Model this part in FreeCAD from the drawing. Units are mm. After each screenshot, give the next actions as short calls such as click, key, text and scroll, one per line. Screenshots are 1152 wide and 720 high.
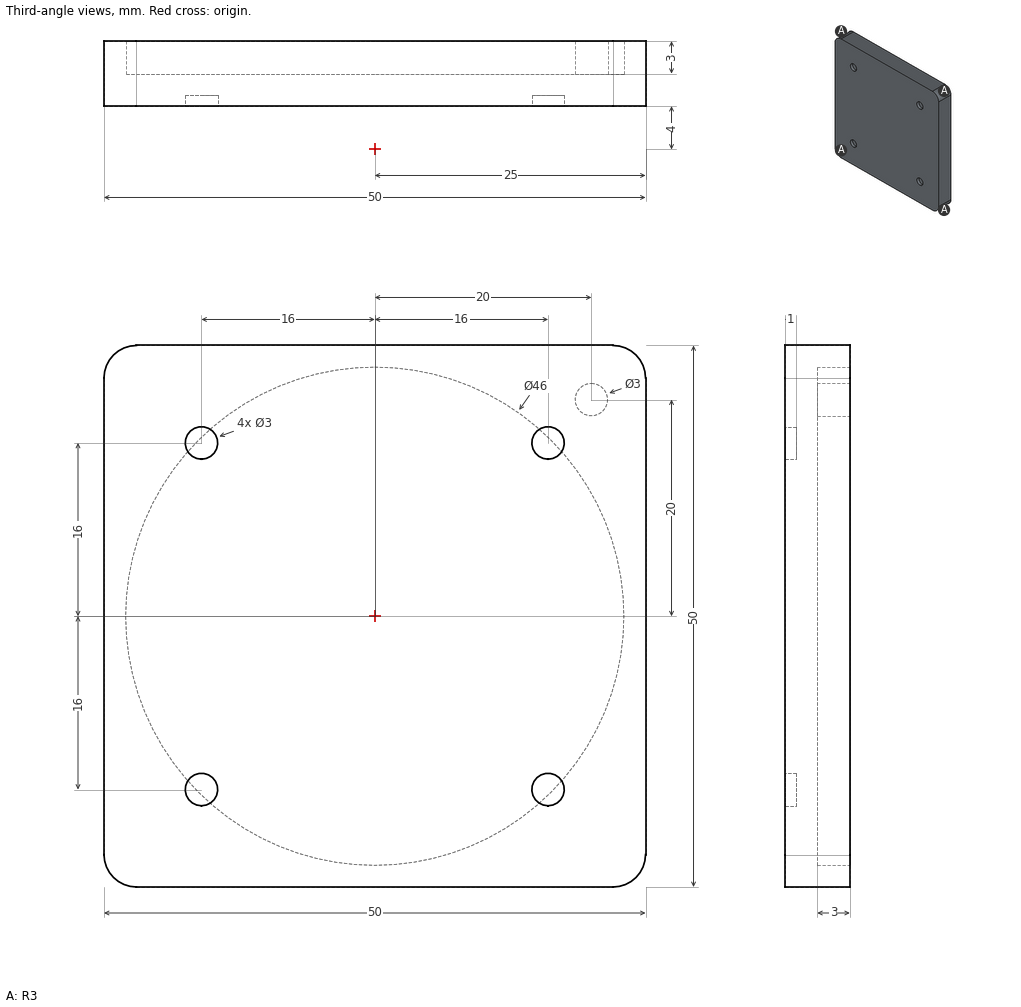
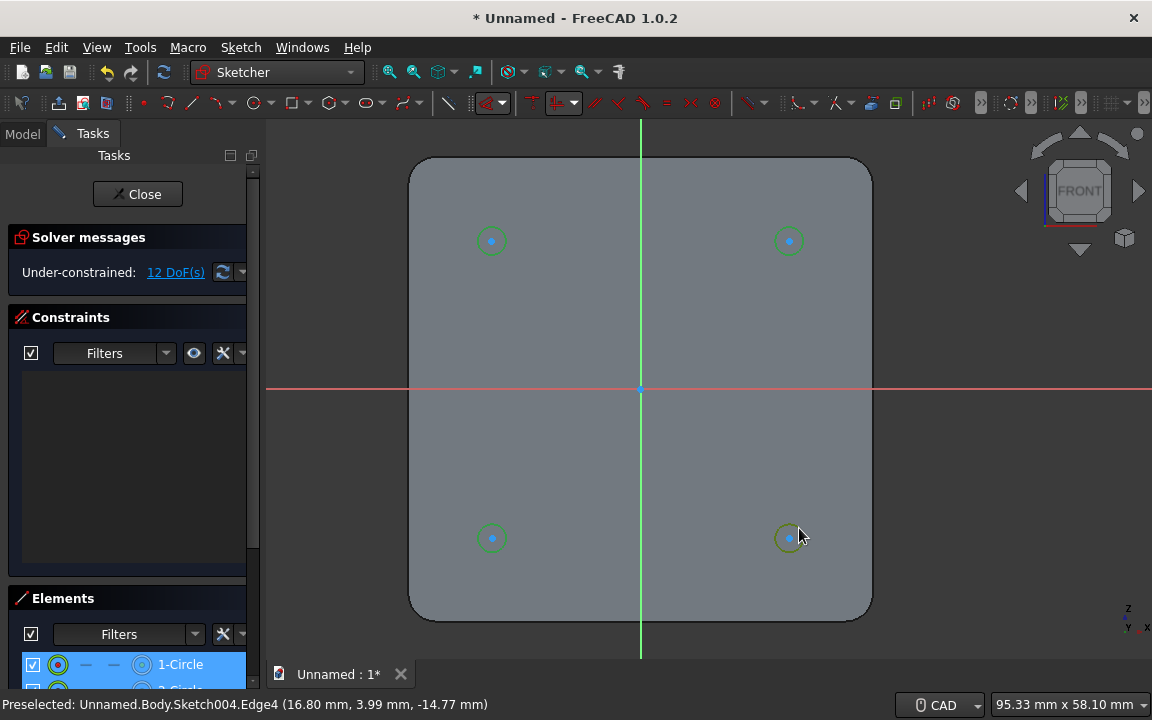
click(668, 104)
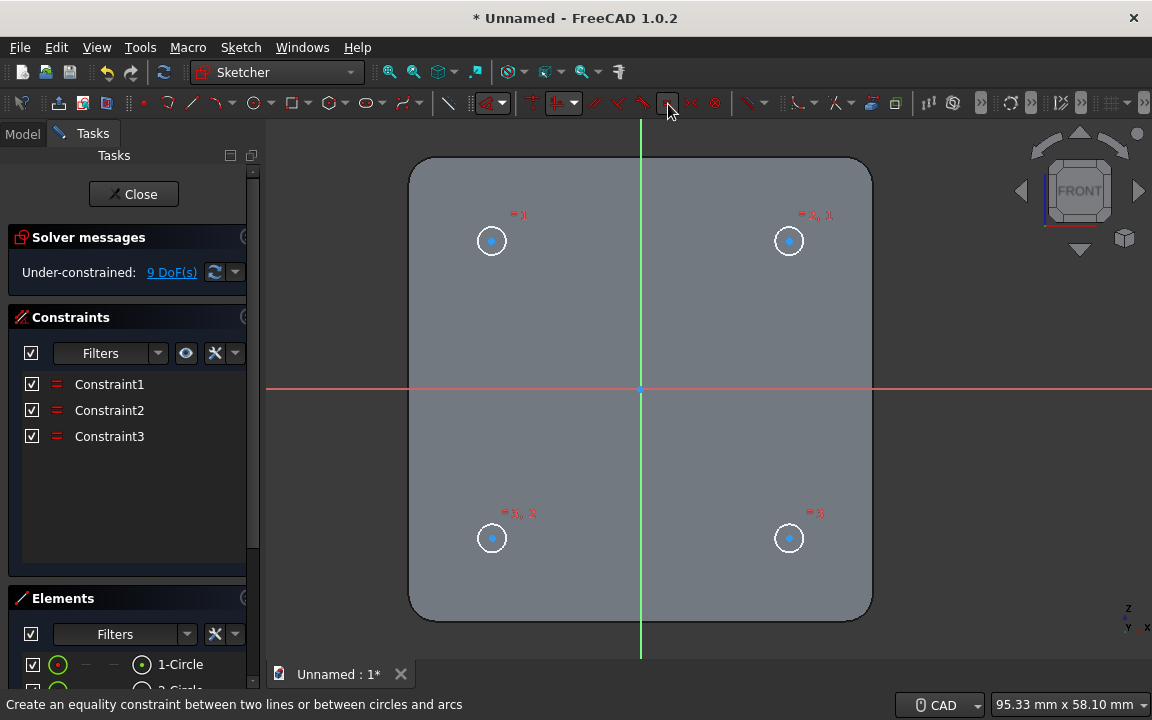
click(492, 241)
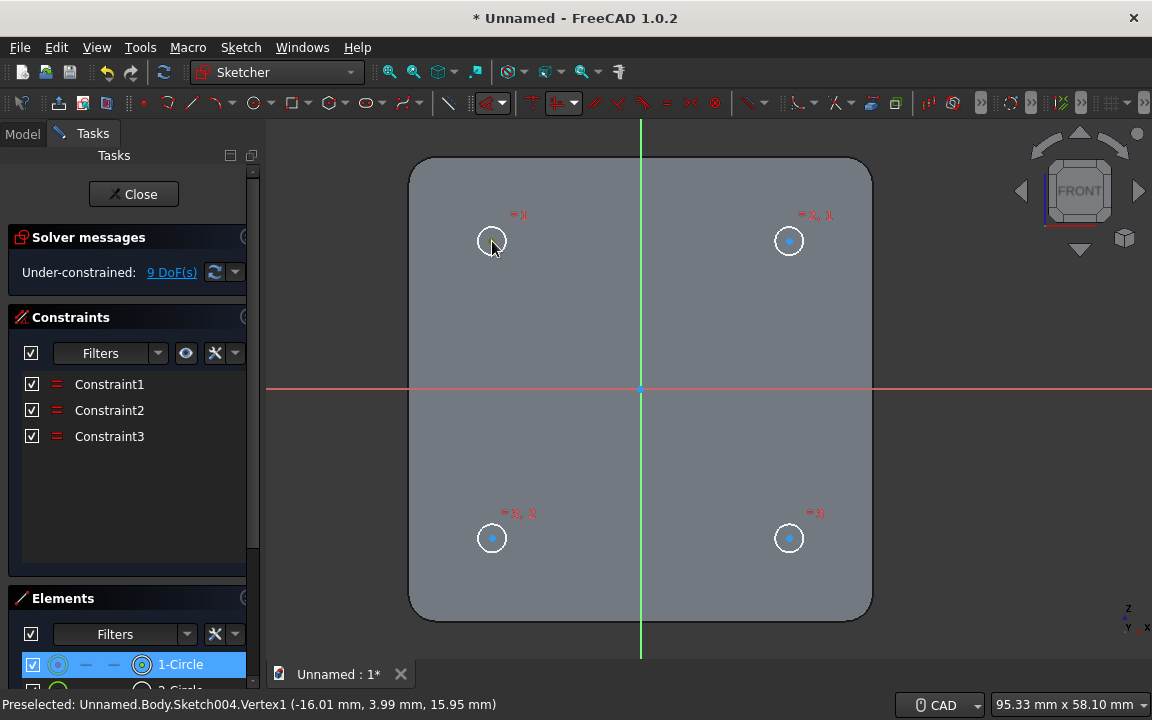
click(789, 241)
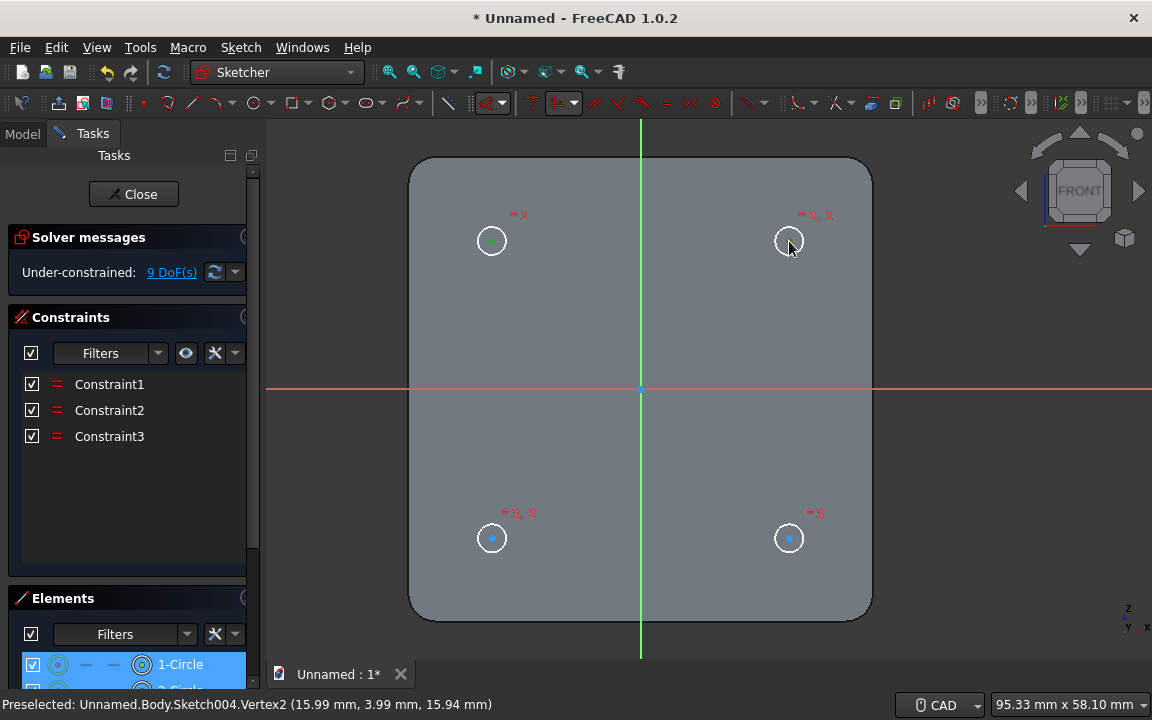
key(h)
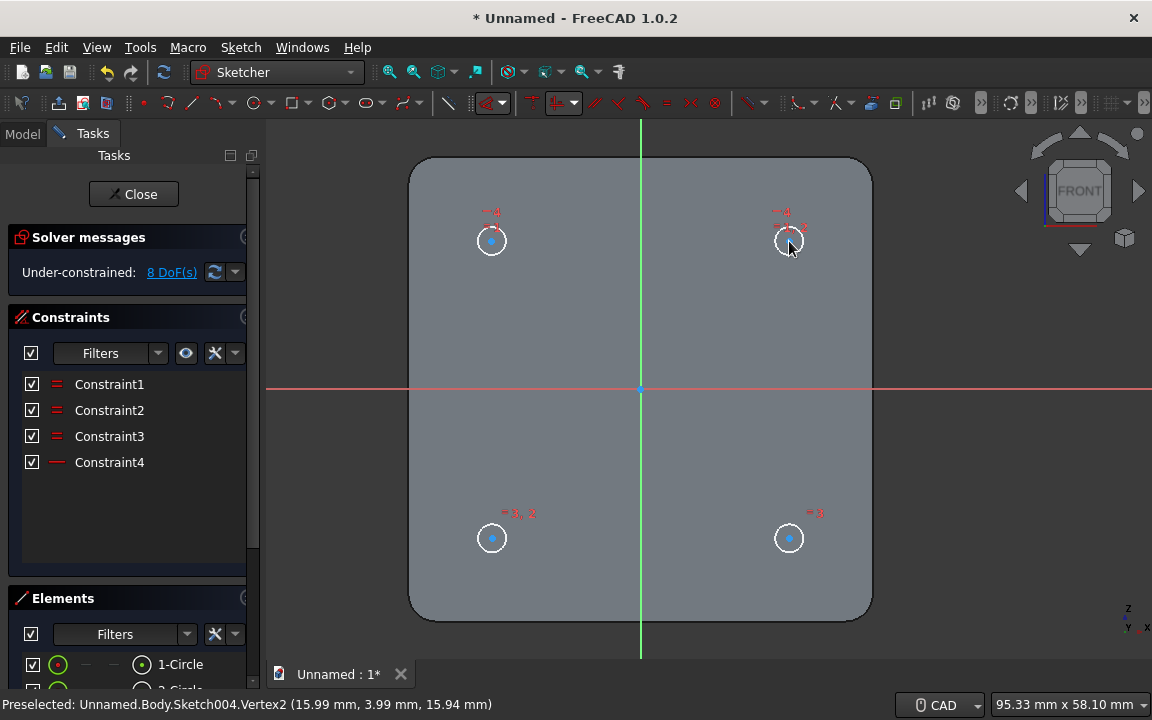
click(492, 241)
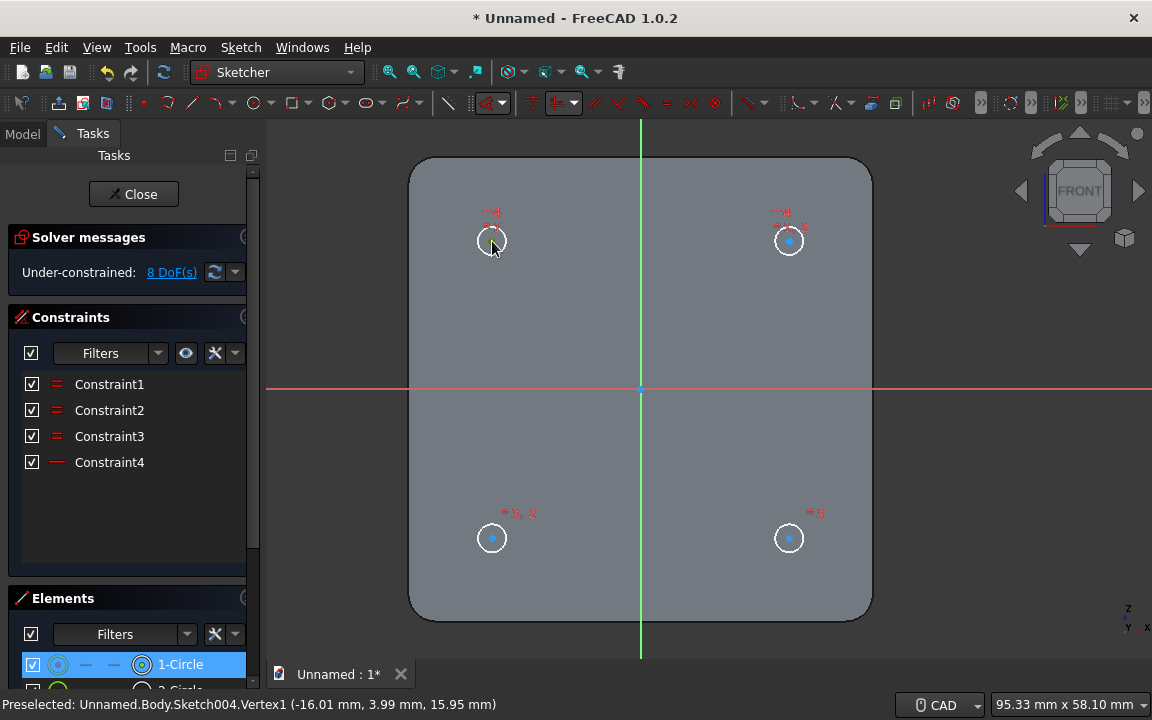
click(492, 538)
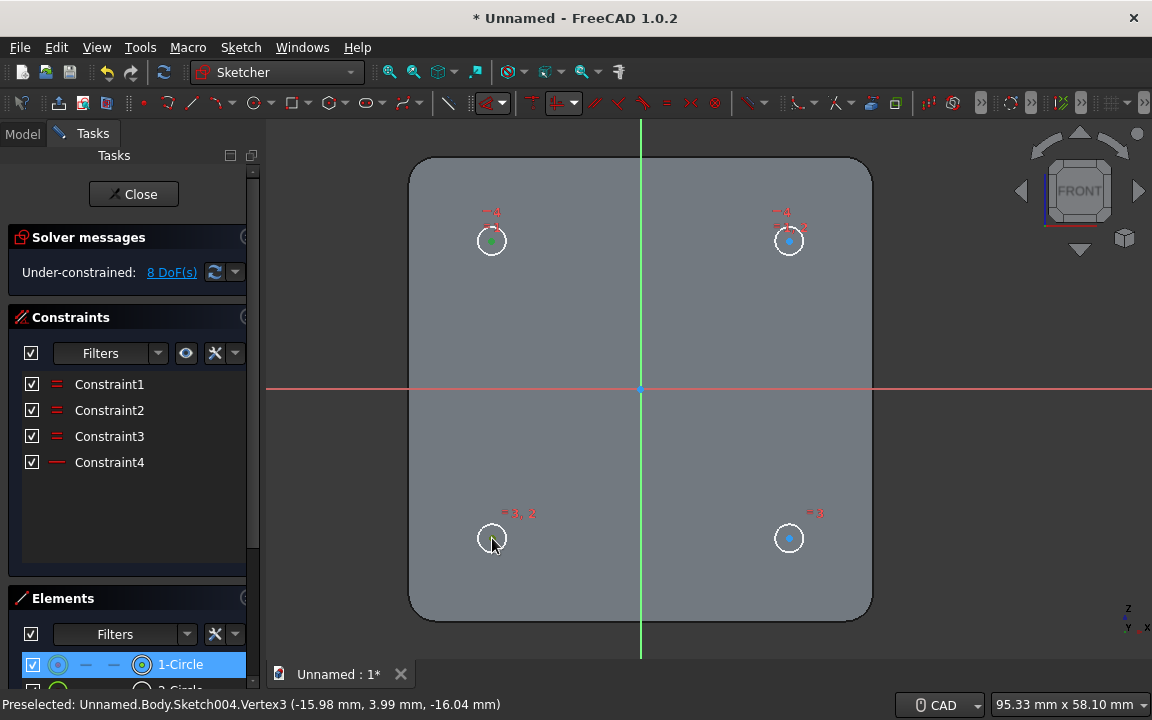
key(v)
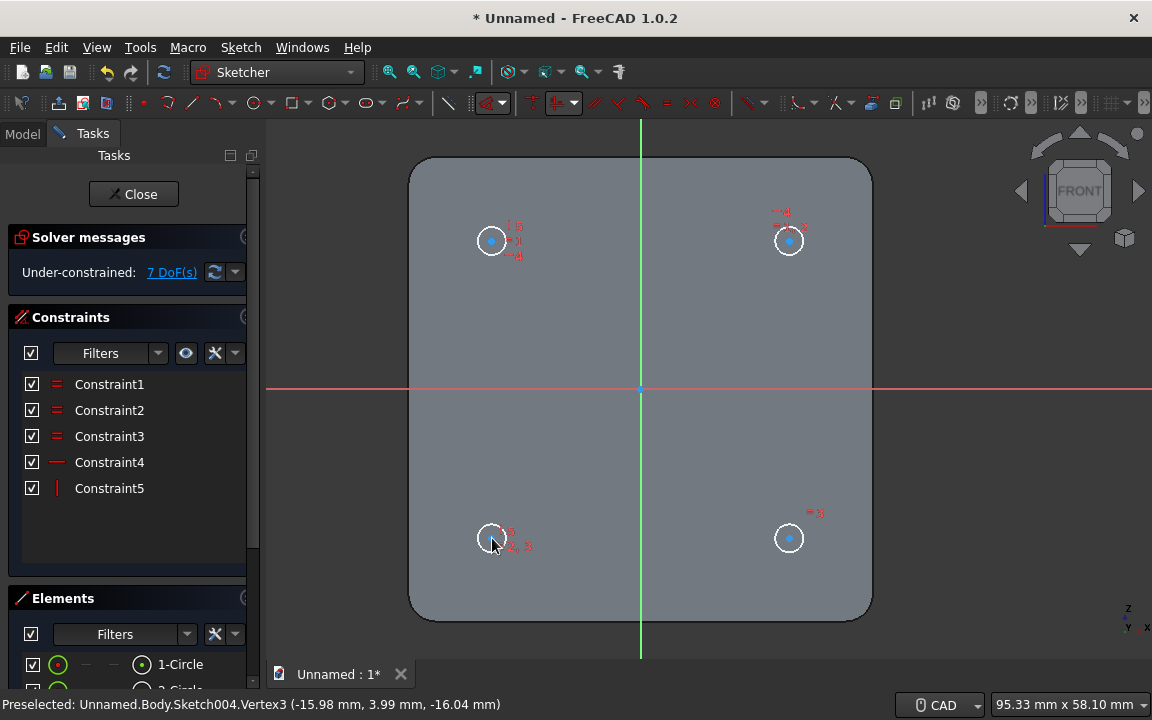
click(789, 241)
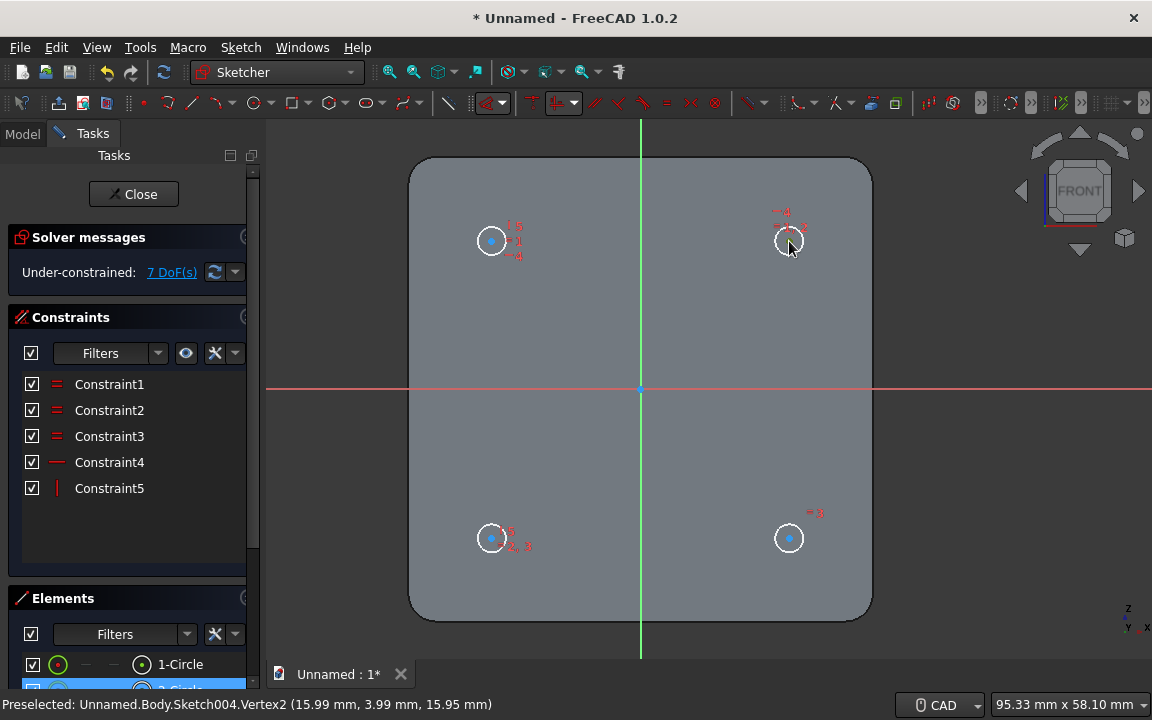
click(789, 538)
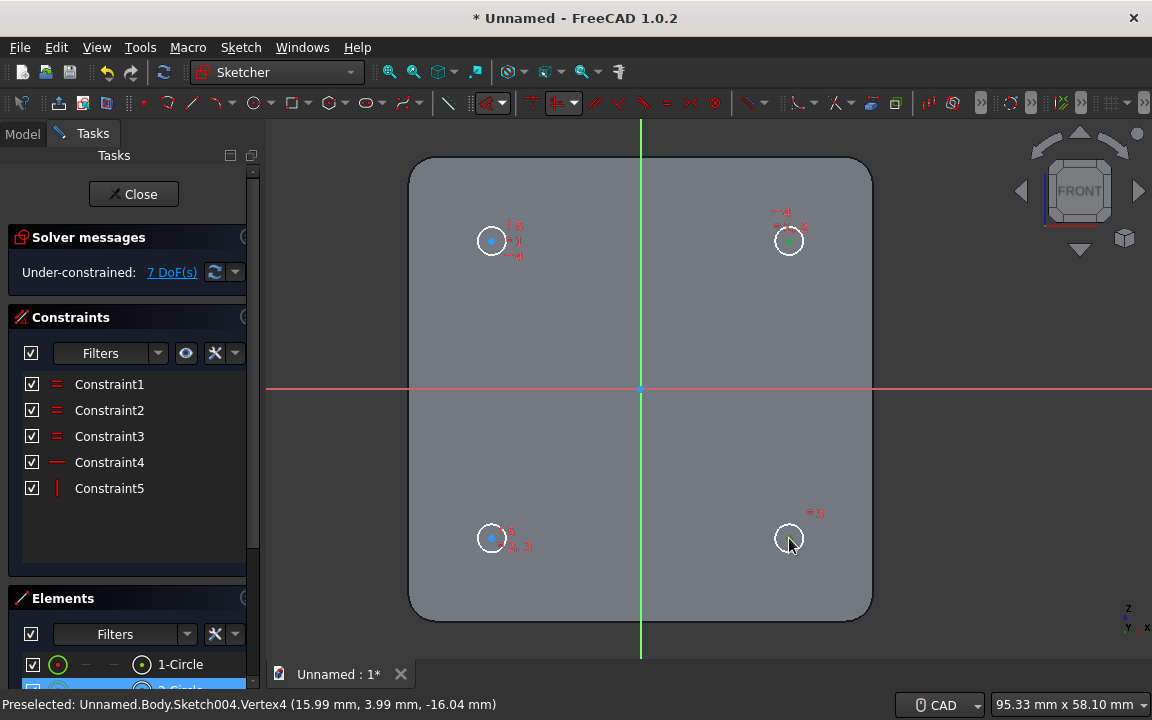
key(v)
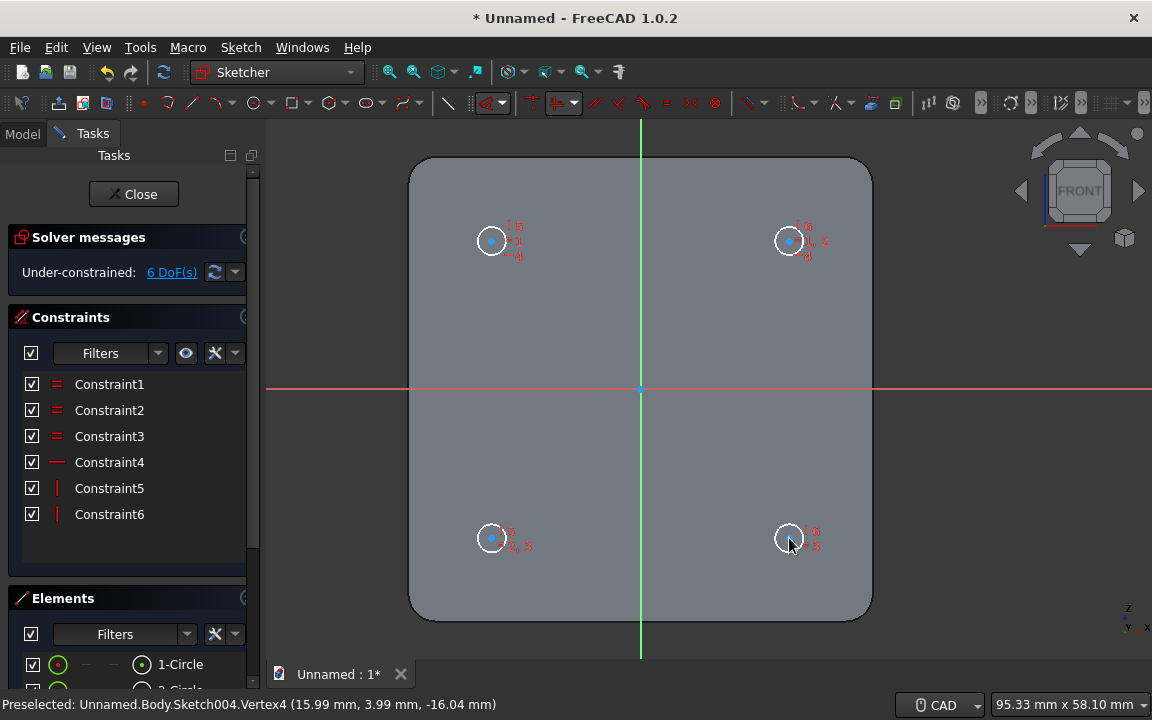
click(492, 538)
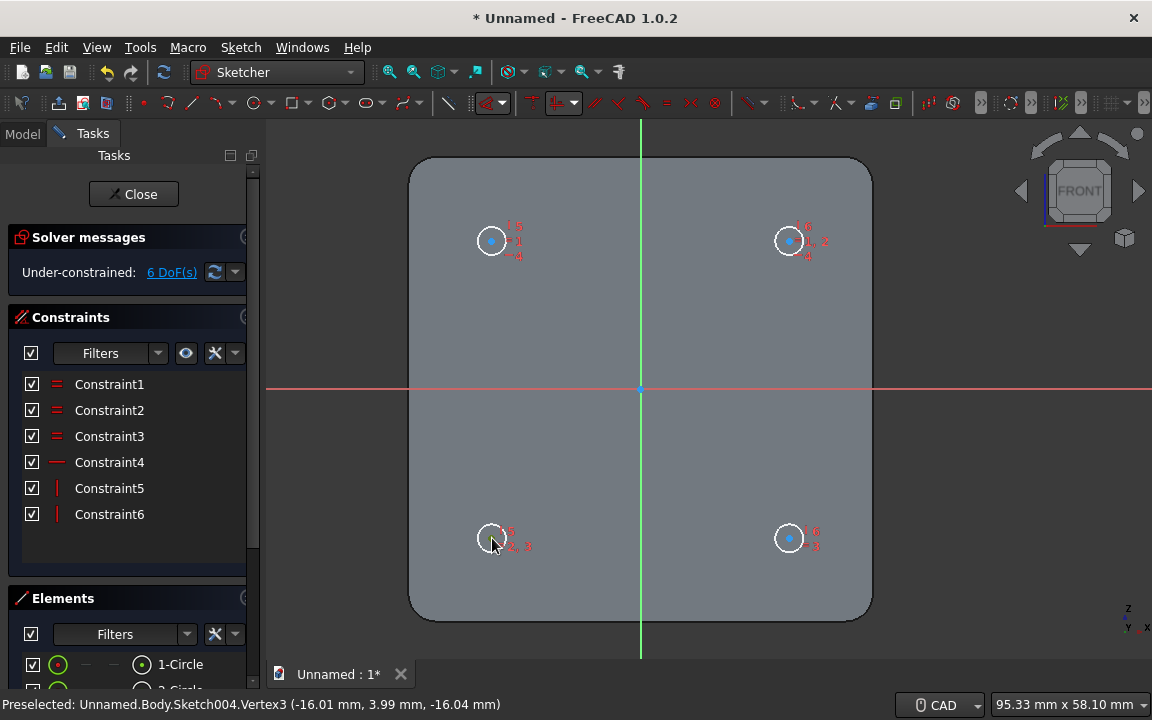
click(789, 538)